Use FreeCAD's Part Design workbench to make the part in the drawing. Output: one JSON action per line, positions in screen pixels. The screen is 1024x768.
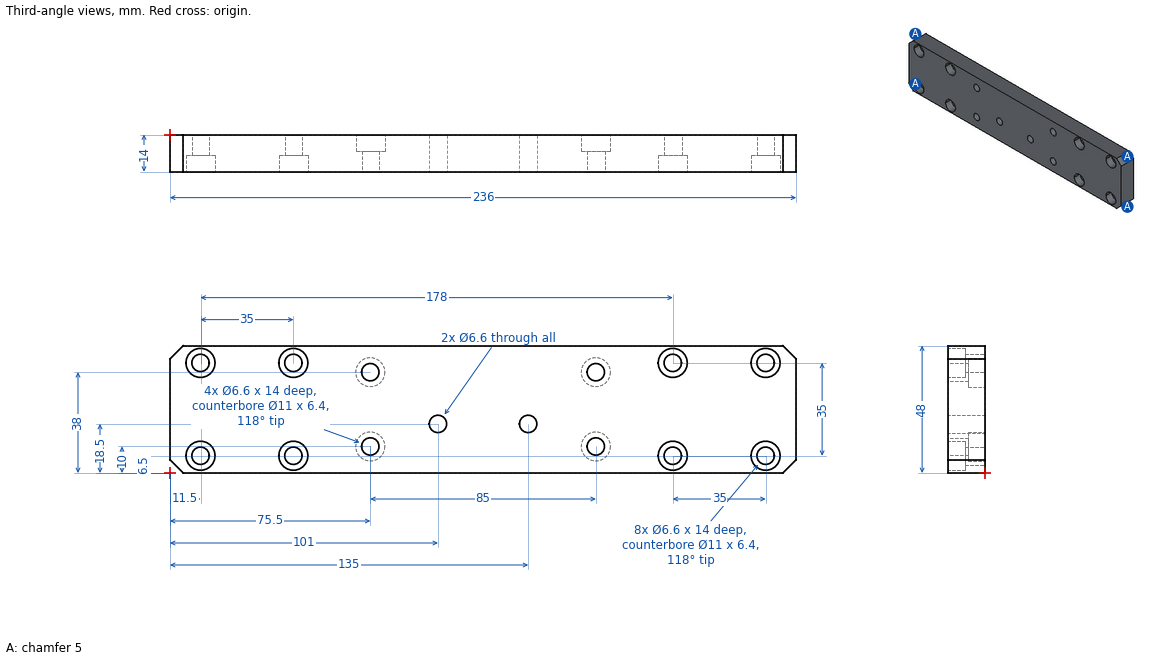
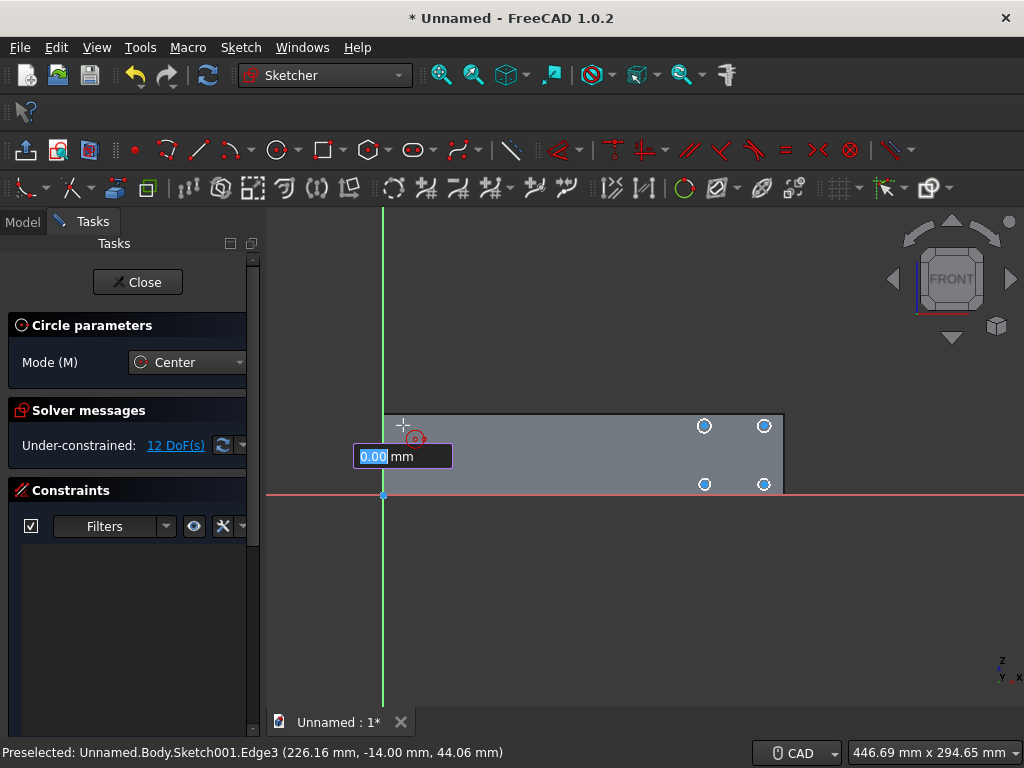
{"action": "scroll", "coordinate": [407, 421], "scroll_direction": "up", "scroll_amount": 6}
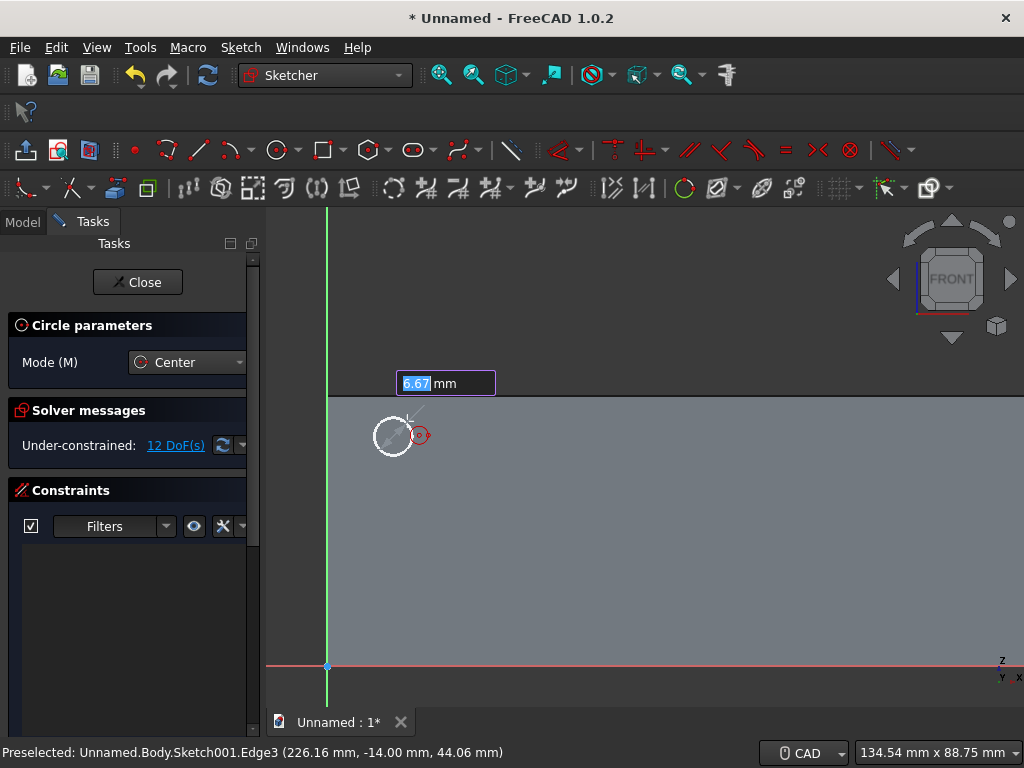
{"action": "left_click", "coordinate": [405, 419]}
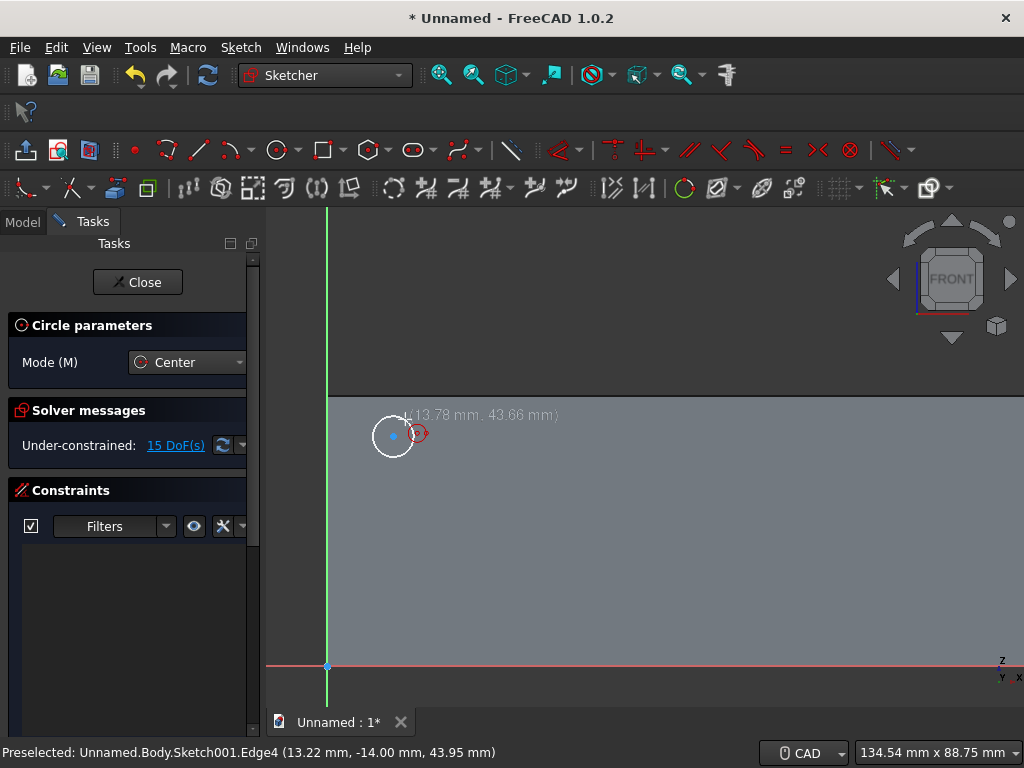
{"action": "left_click", "coordinate": [589, 432]}
{"action": "left_click", "coordinate": [602, 419]}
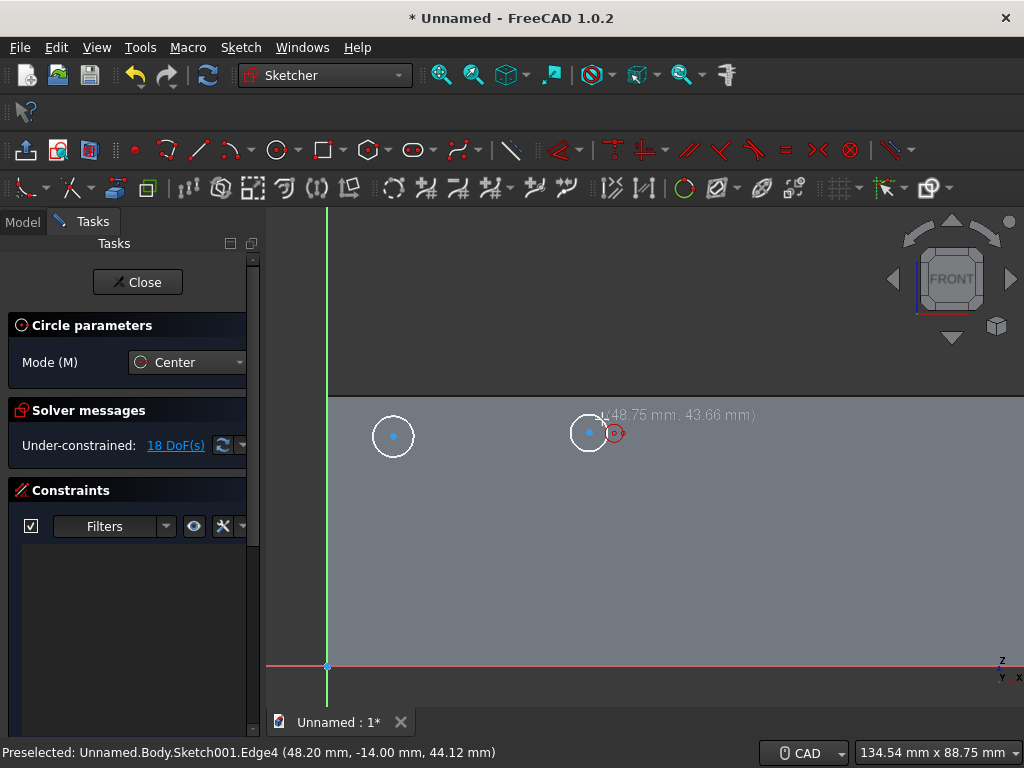
{"action": "left_click", "coordinate": [589, 629]}
{"action": "left_click", "coordinate": [602, 616]}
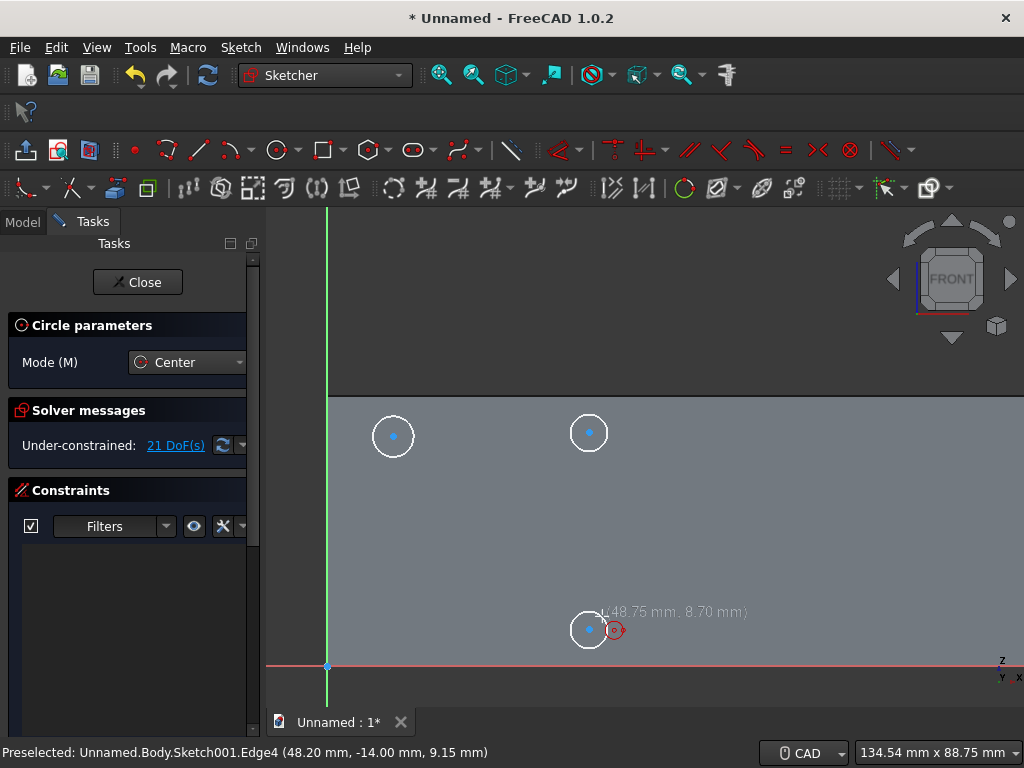
{"action": "left_click", "coordinate": [392, 629]}
{"action": "left_click", "coordinate": [405, 616]}
{"action": "key", "text": "Escape"}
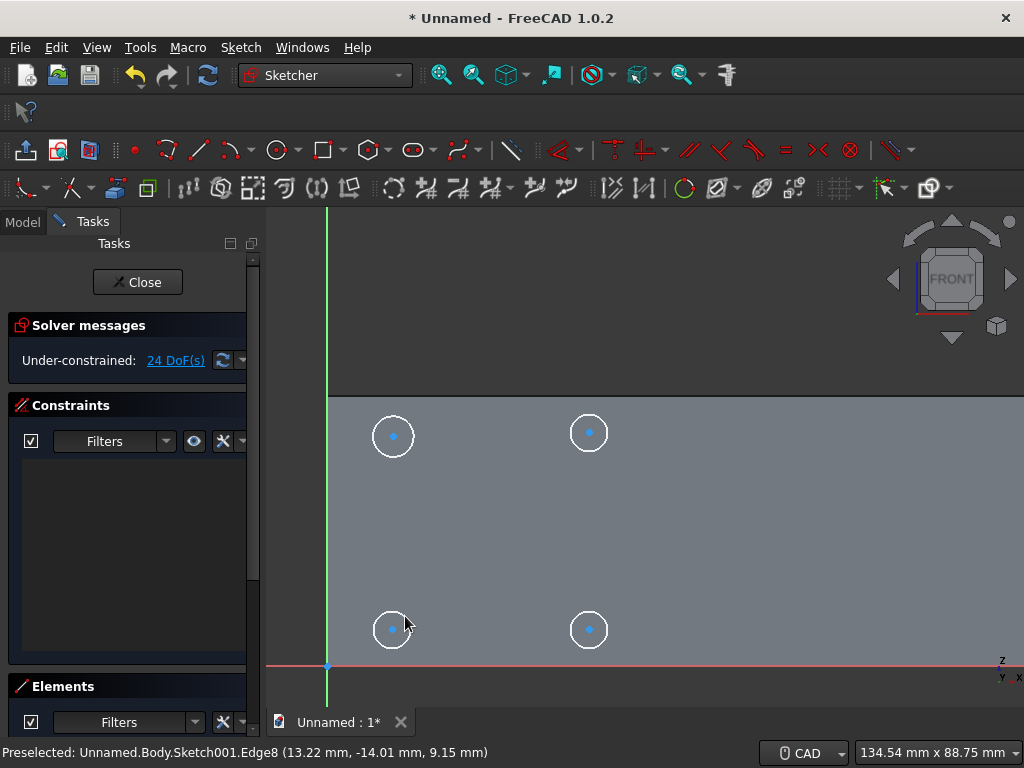
{"action": "scroll", "coordinate": [407, 421], "scroll_direction": "down", "scroll_amount": 6}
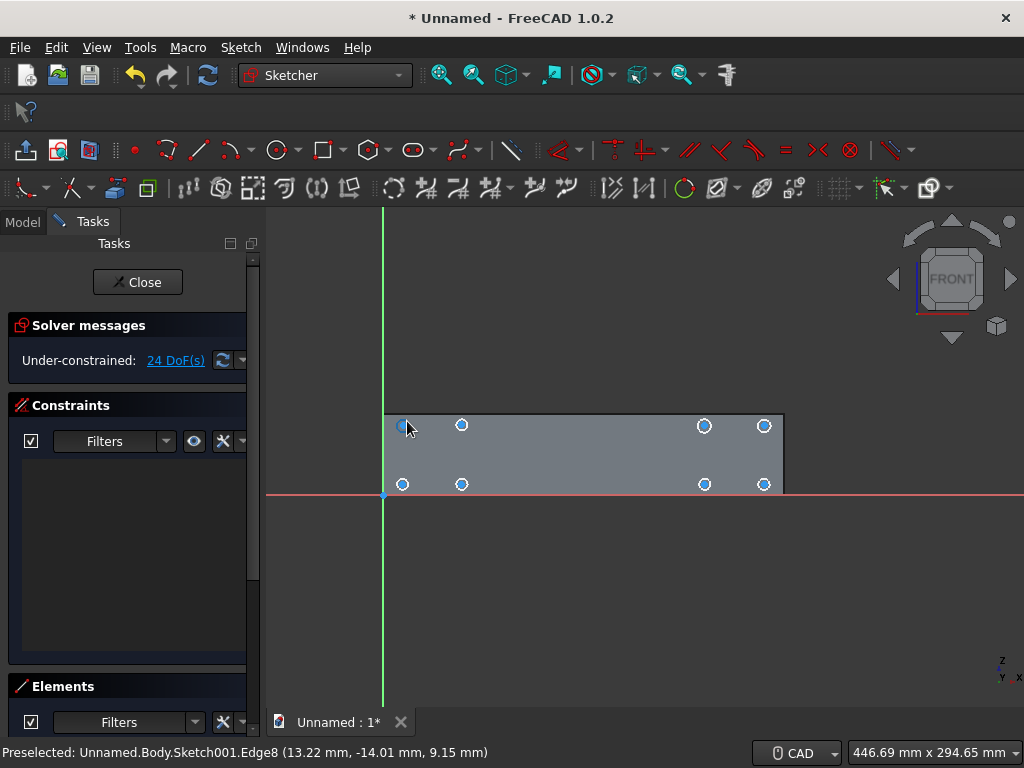
{"action": "scroll", "coordinate": [768, 480], "scroll_direction": "up", "scroll_amount": 5}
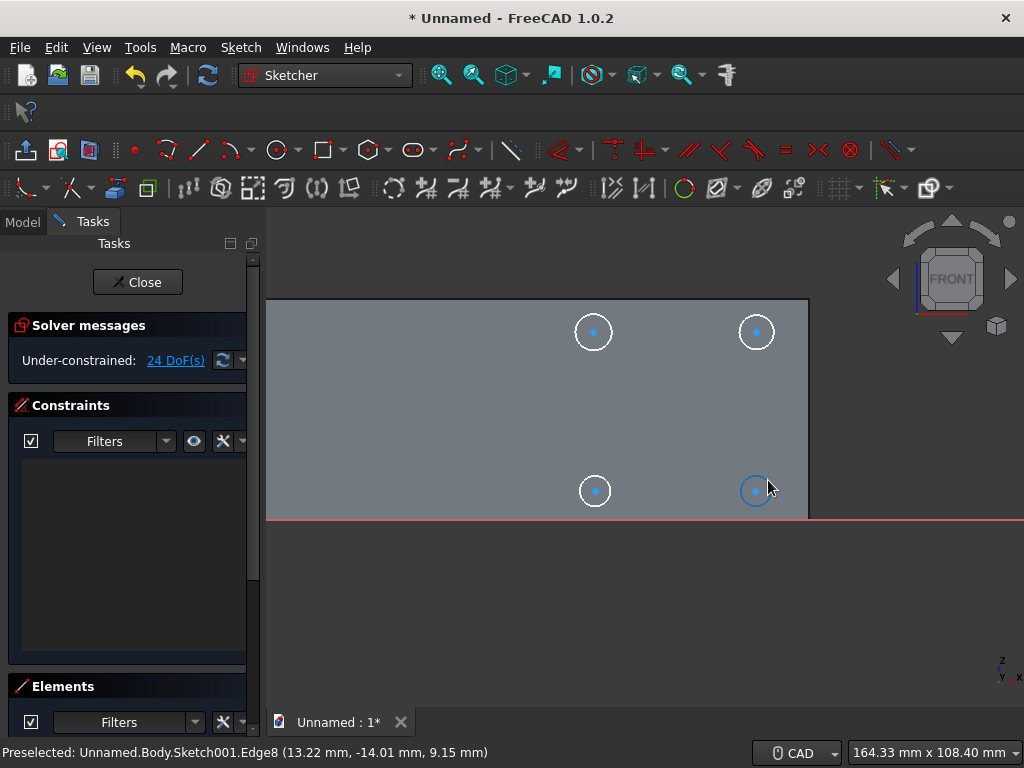
{"action": "left_click", "coordinate": [767, 480]}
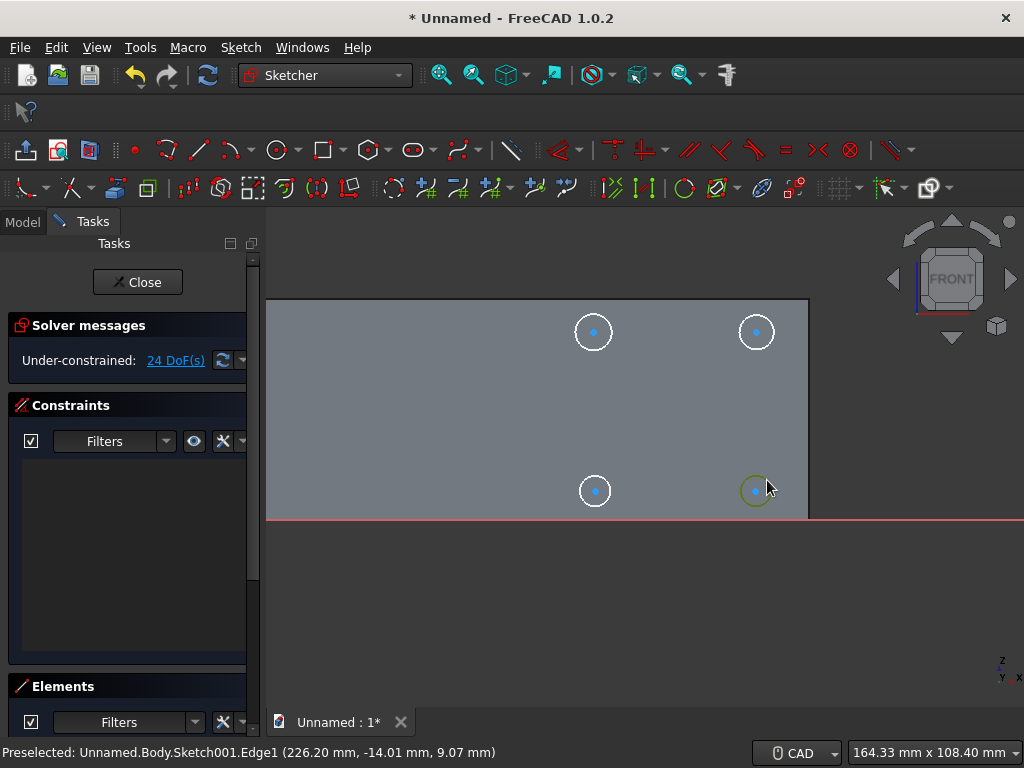
{"action": "left_click", "coordinate": [606, 480]}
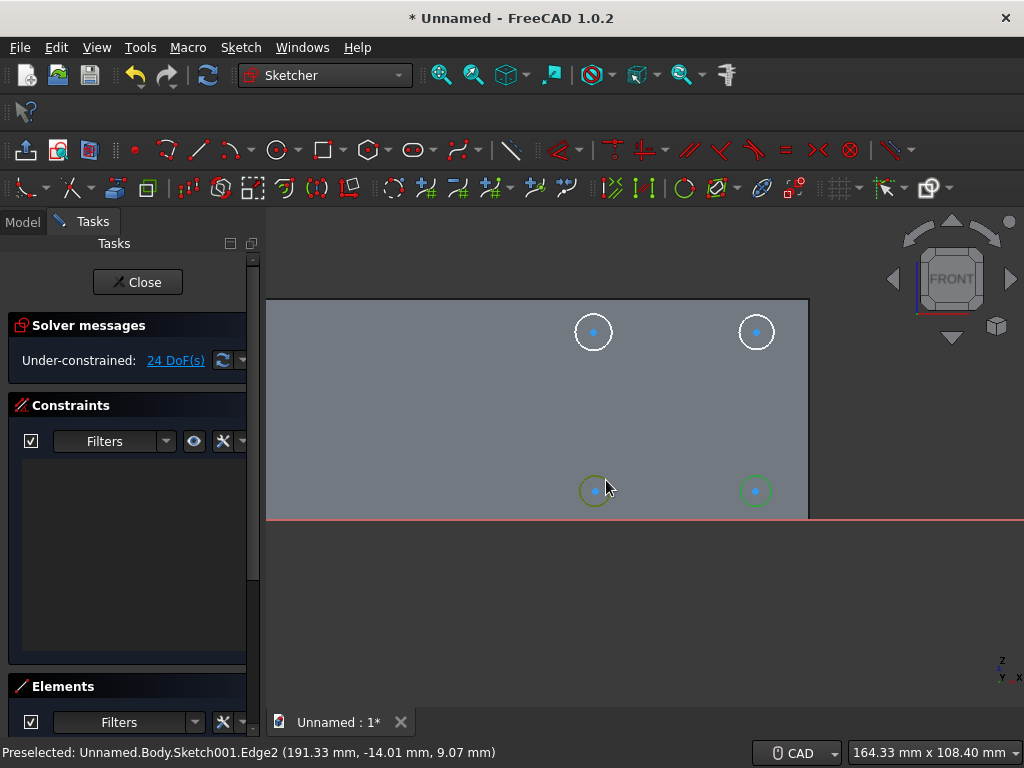
{"action": "left_click", "coordinate": [606, 319]}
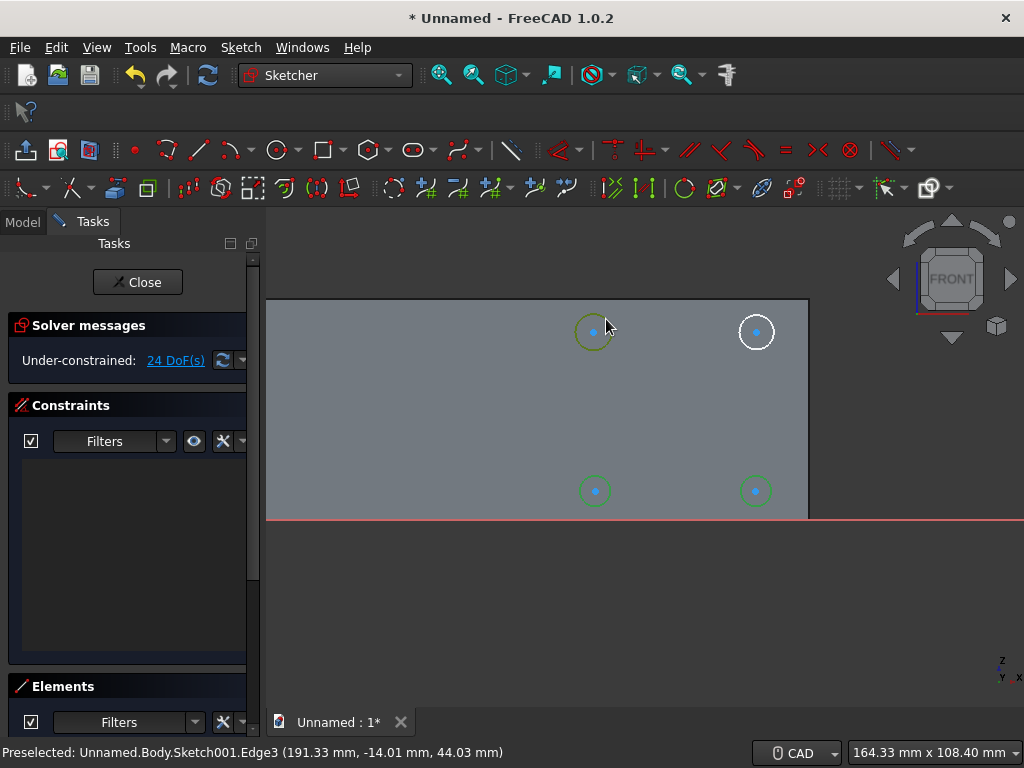
{"action": "left_click", "coordinate": [769, 320]}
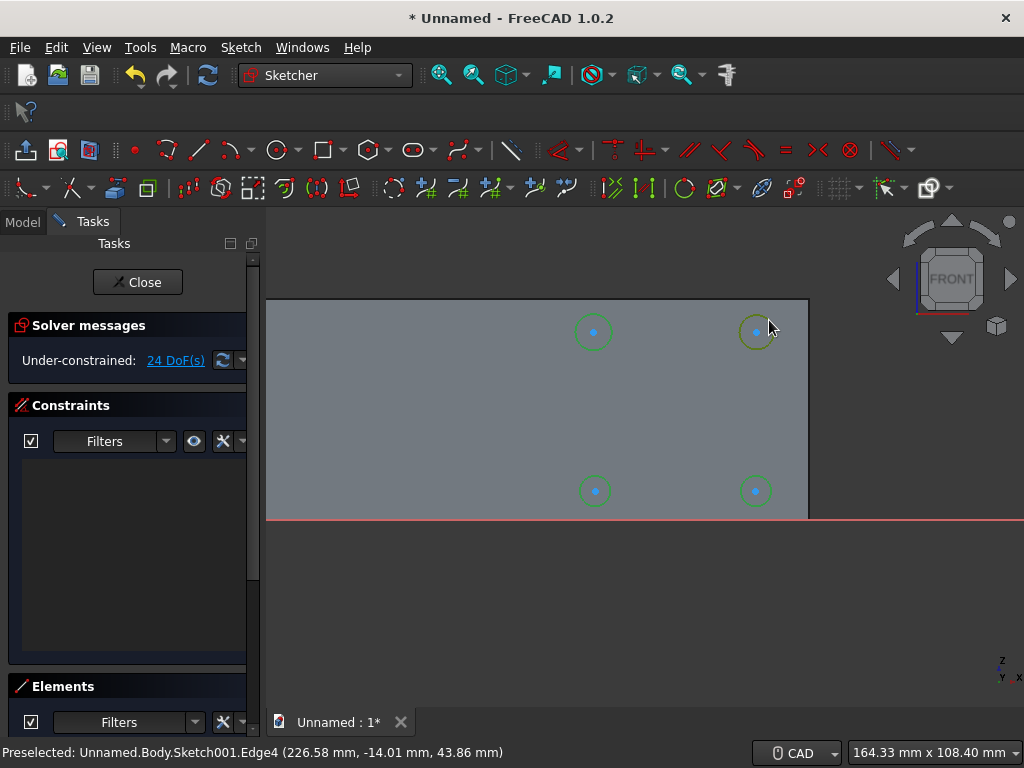
{"action": "scroll", "coordinate": [769, 480], "scroll_direction": "down", "scroll_amount": 5}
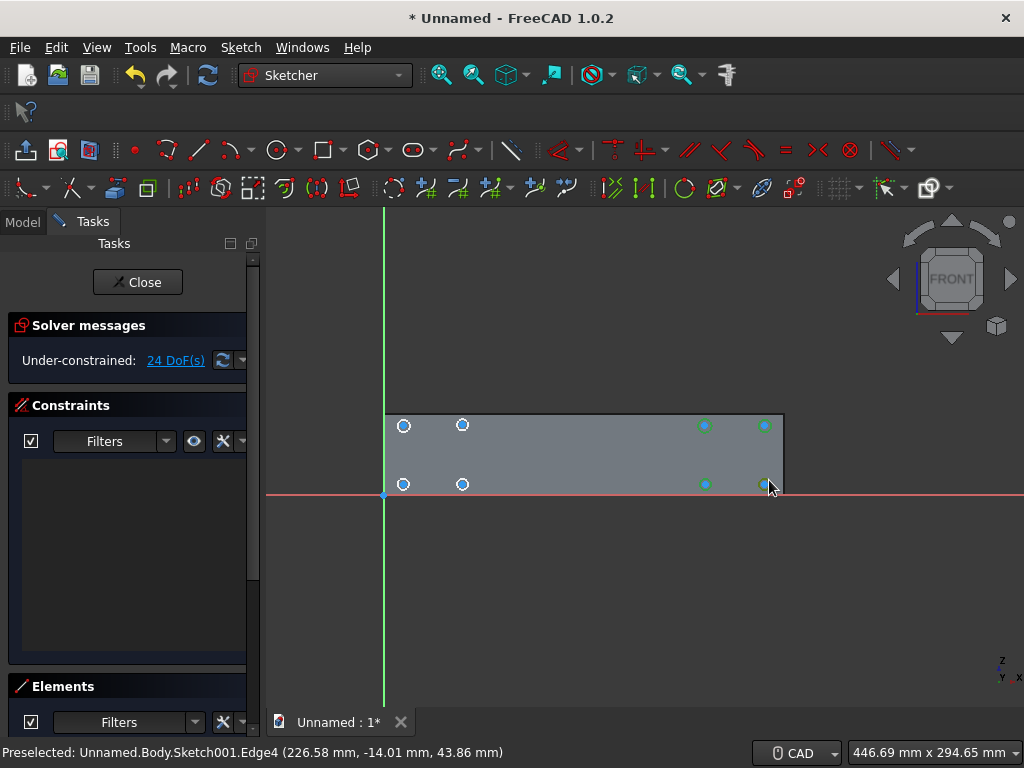
{"action": "scroll", "coordinate": [408, 422], "scroll_direction": "up", "scroll_amount": 5}